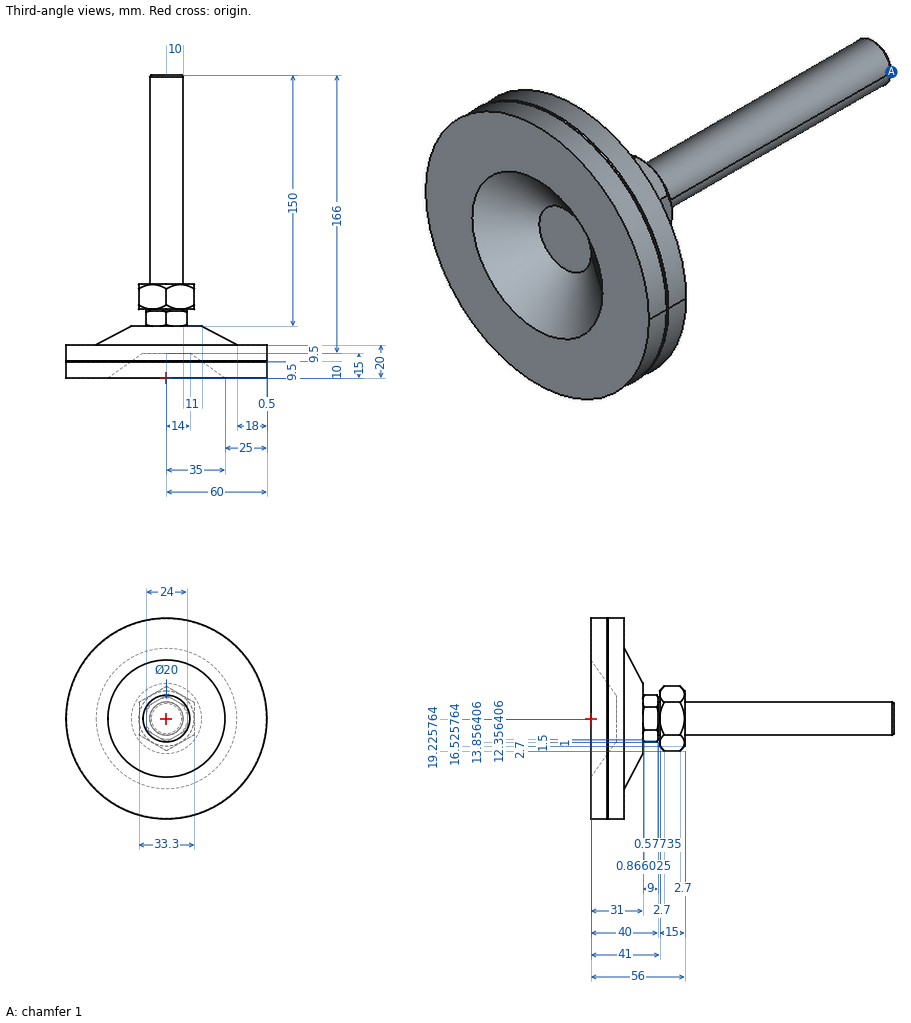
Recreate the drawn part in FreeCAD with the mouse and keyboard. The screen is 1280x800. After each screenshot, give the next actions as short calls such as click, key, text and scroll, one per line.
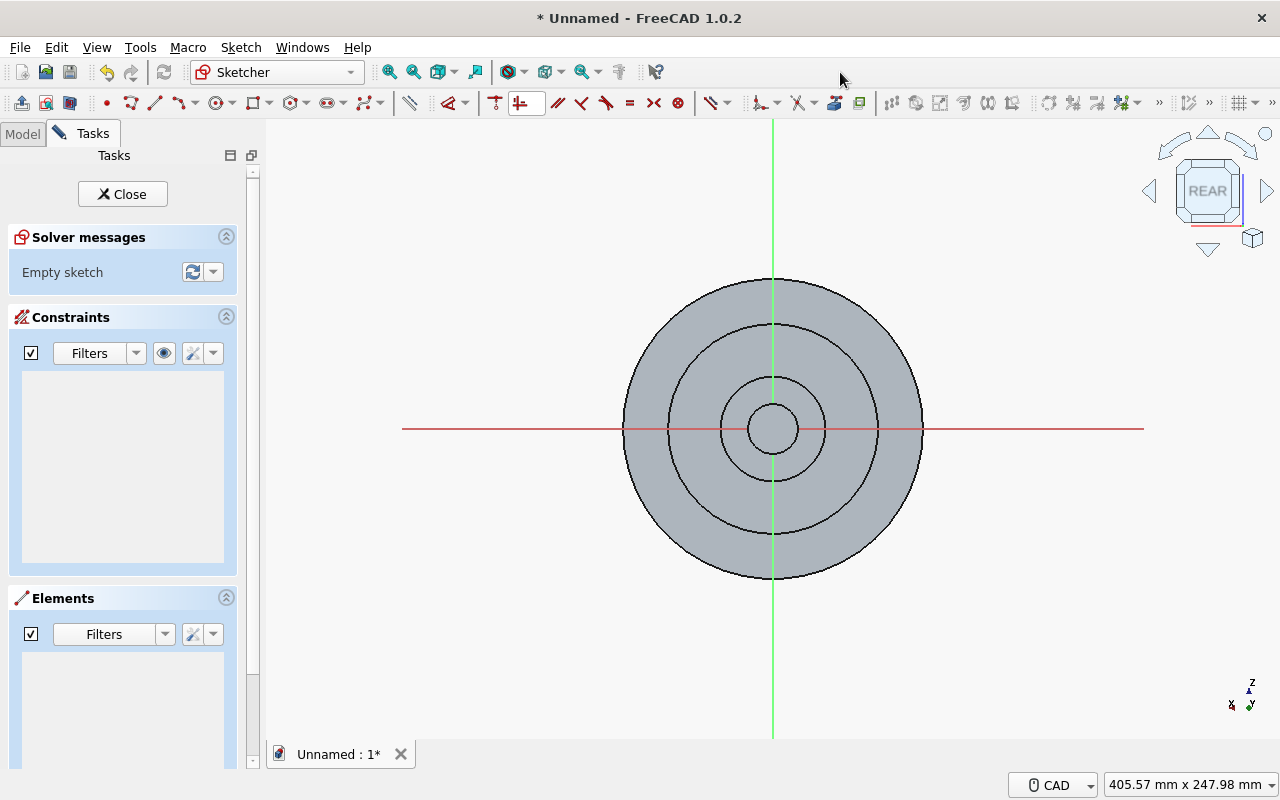
click(70, 104)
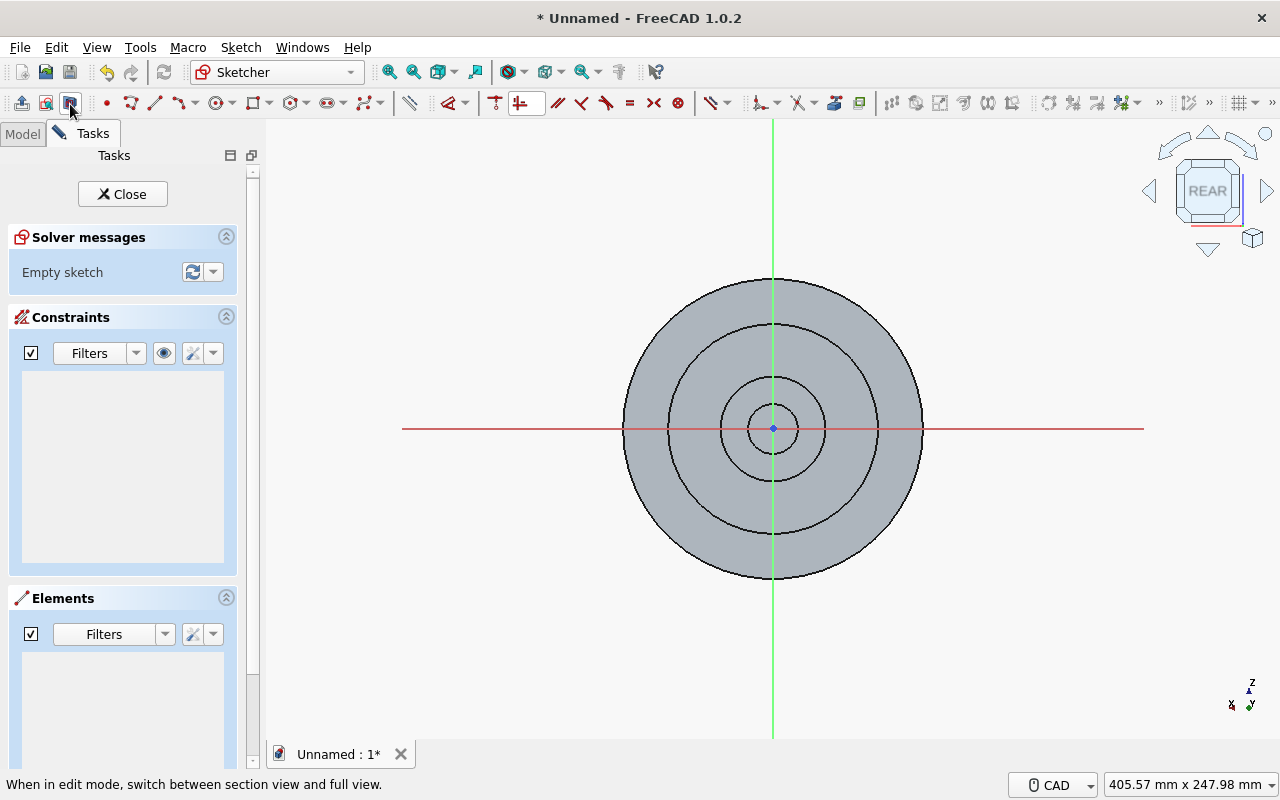
scroll(787, 429, up, 9)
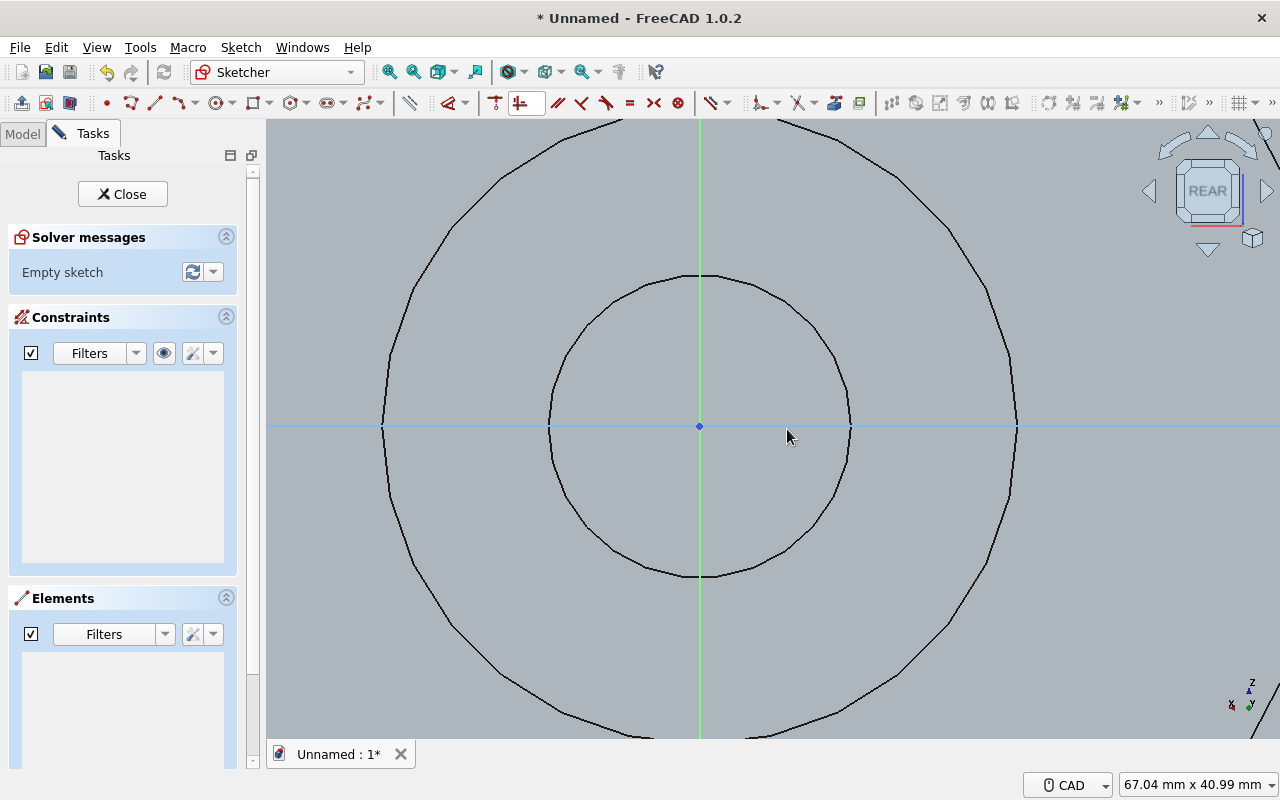
click(290, 104)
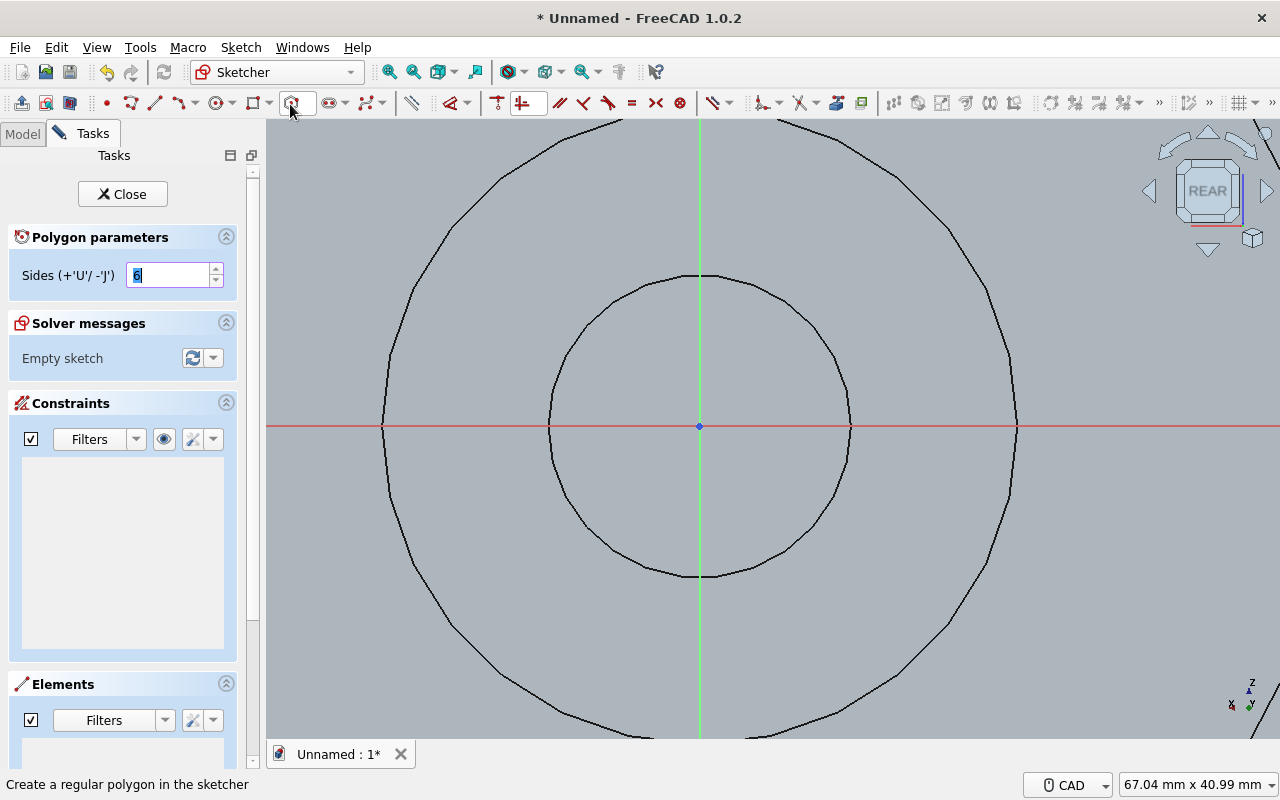
click(700, 426)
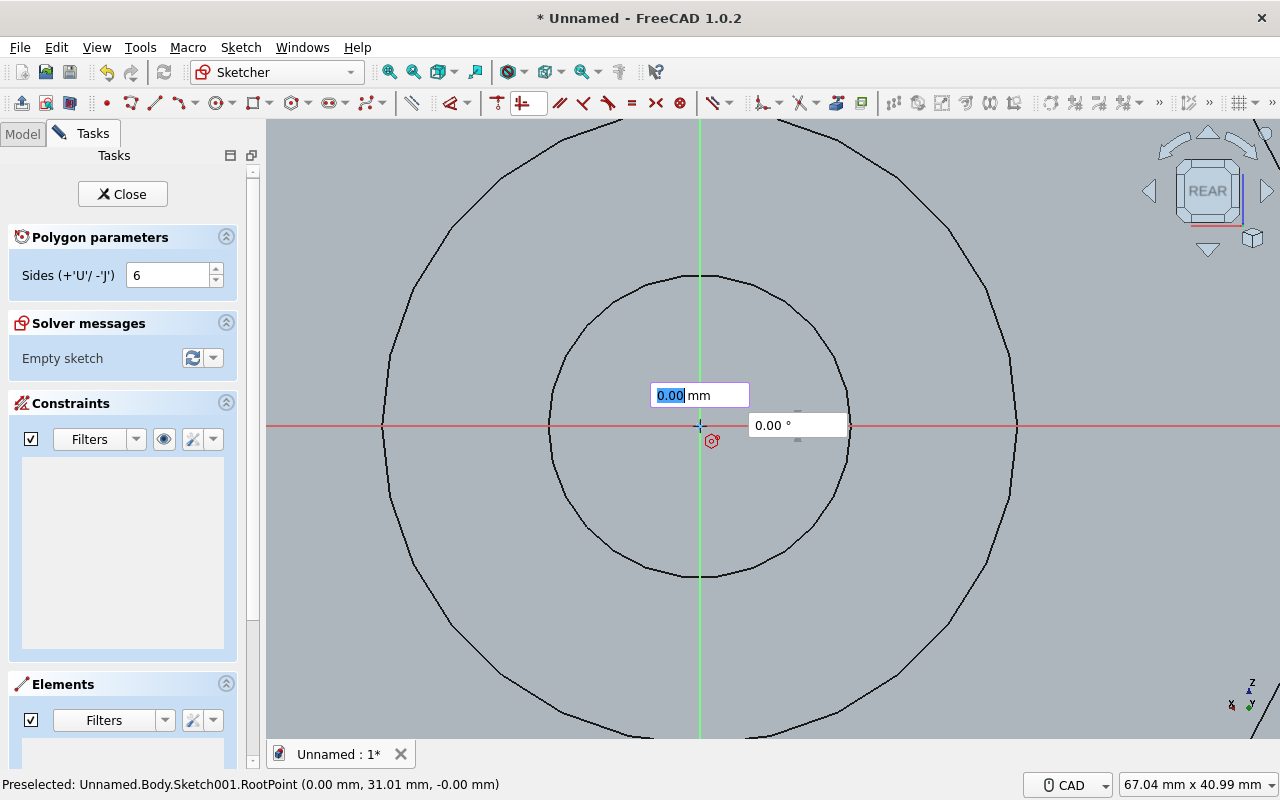
click(700, 636)
right_click(700, 636)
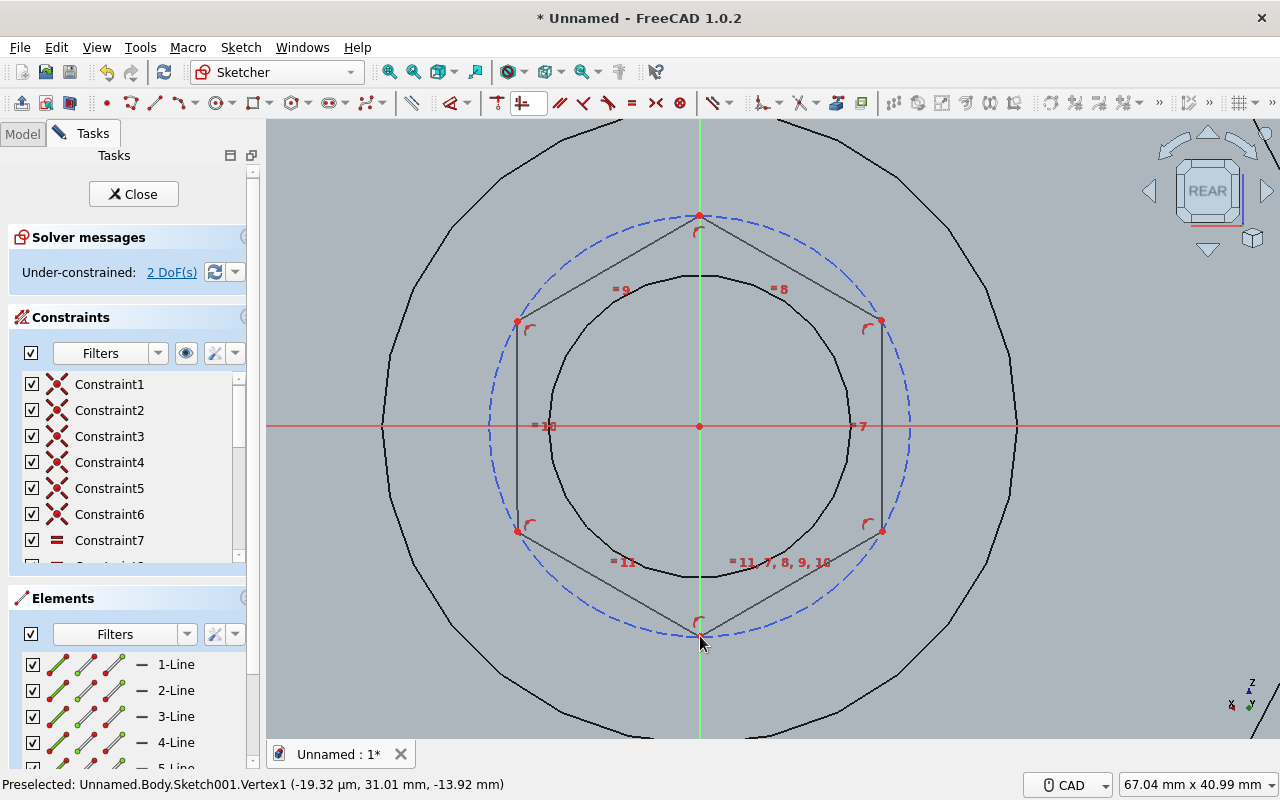
click(882, 468)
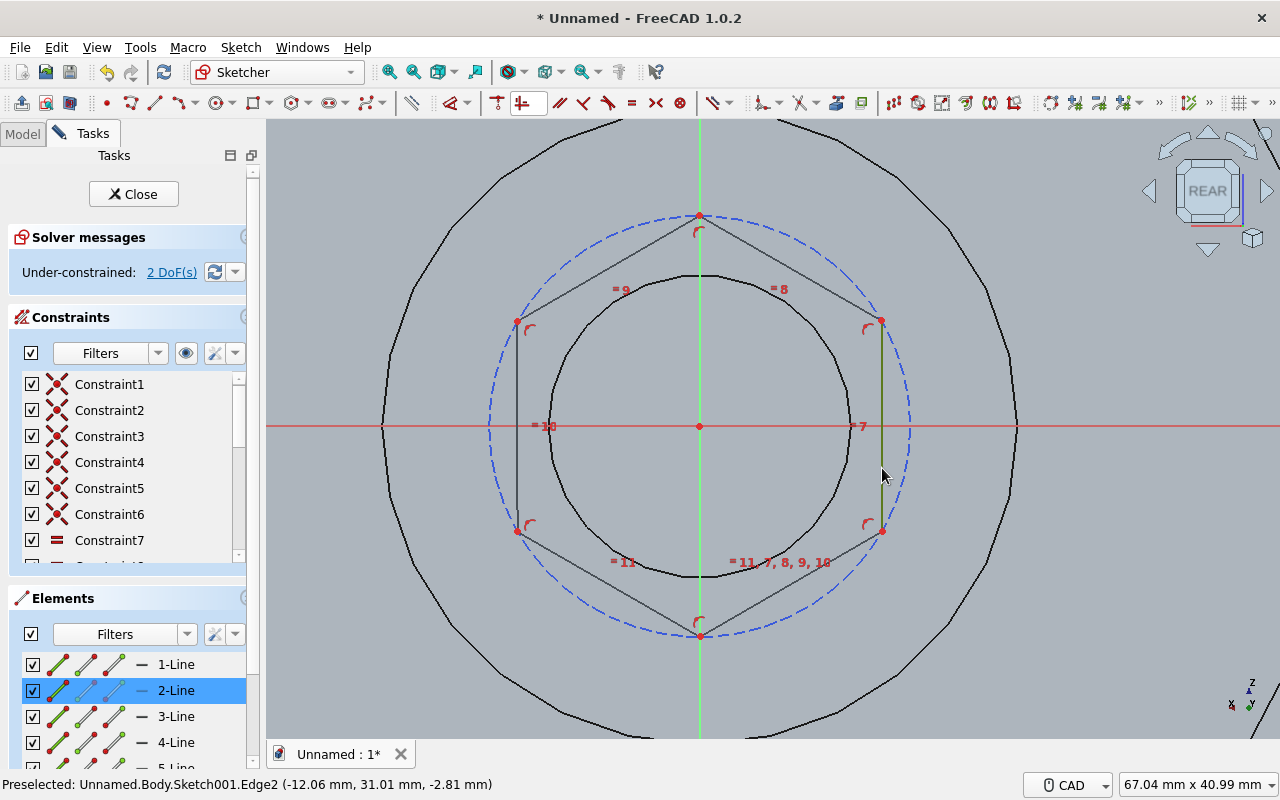
click(542, 104)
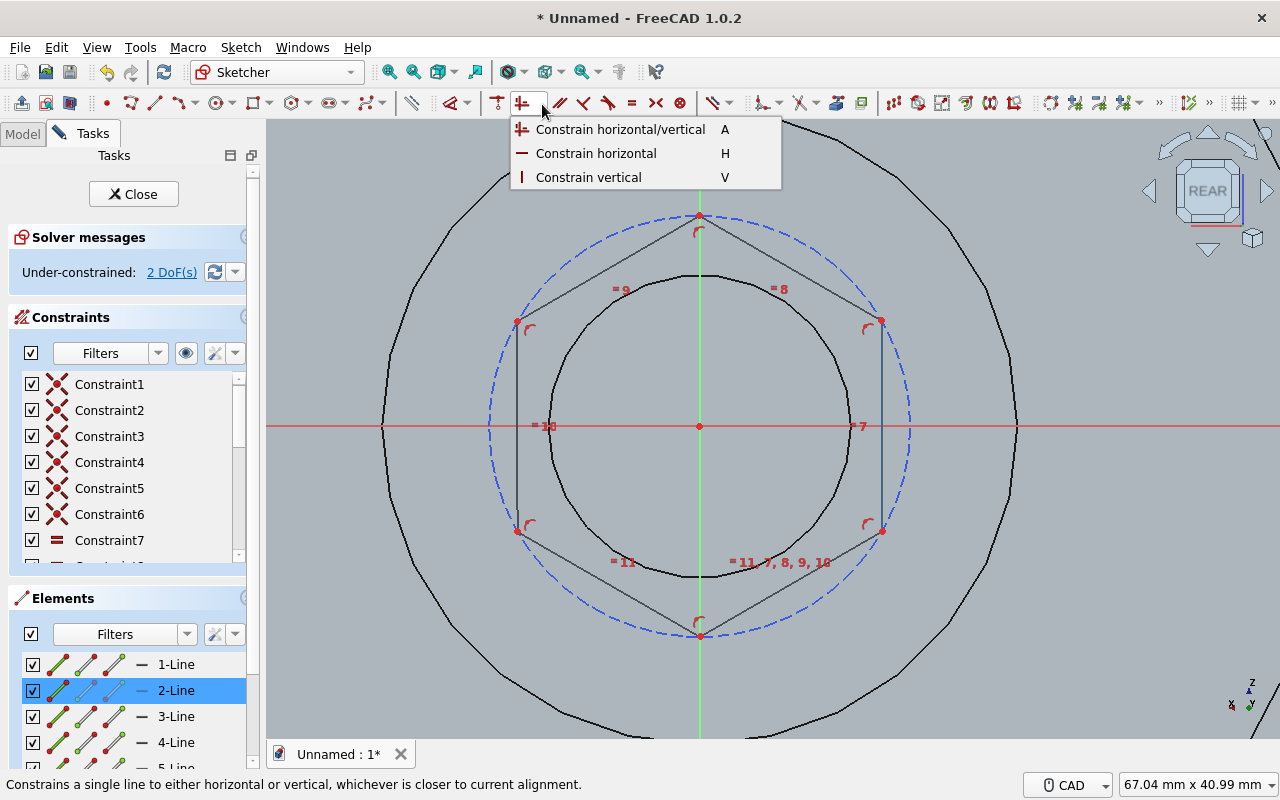
click(646, 177)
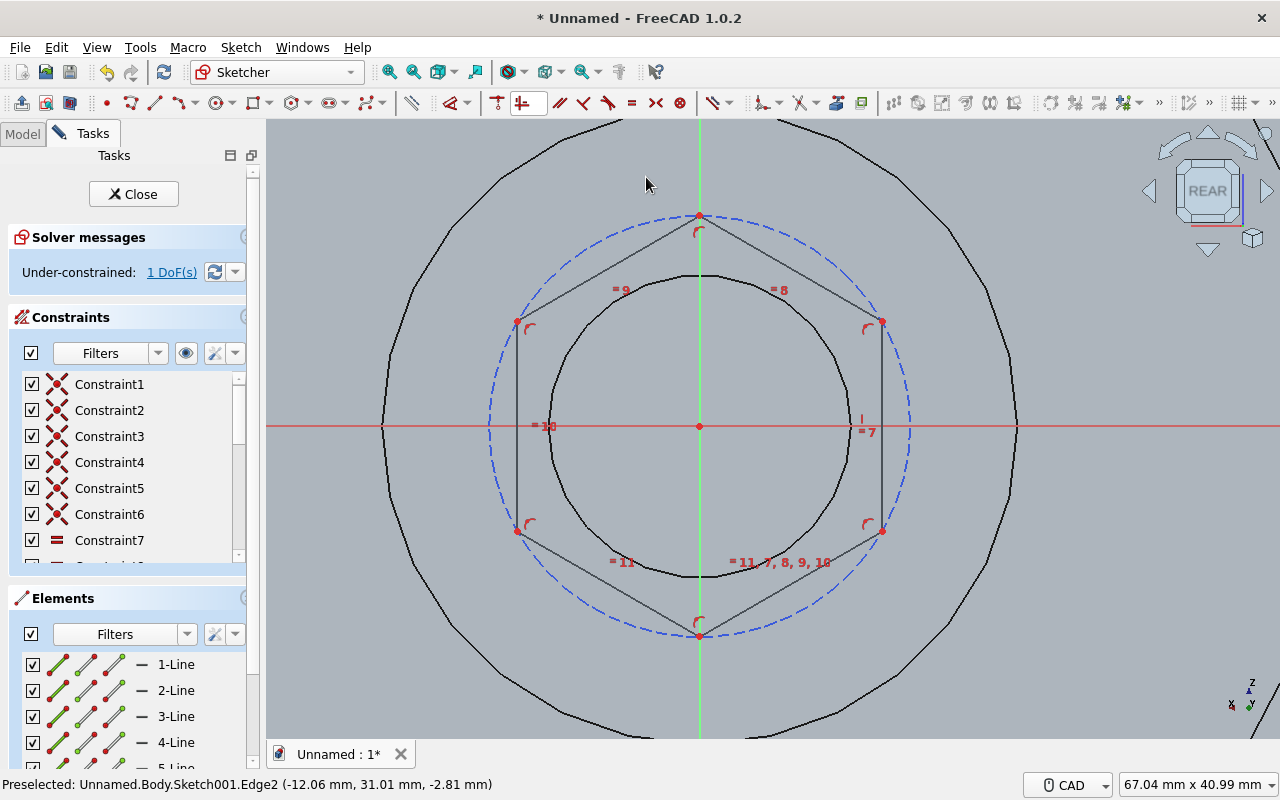
click(450, 104)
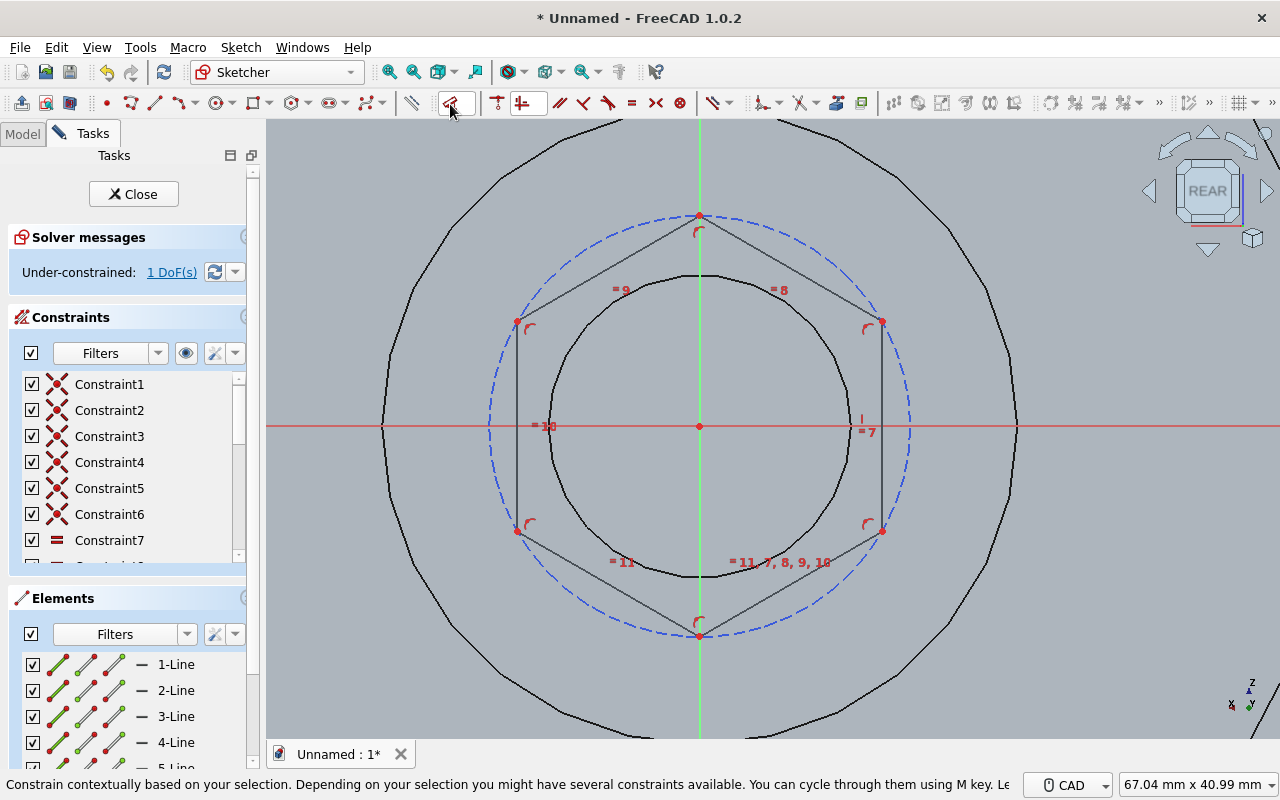
click(517, 321)